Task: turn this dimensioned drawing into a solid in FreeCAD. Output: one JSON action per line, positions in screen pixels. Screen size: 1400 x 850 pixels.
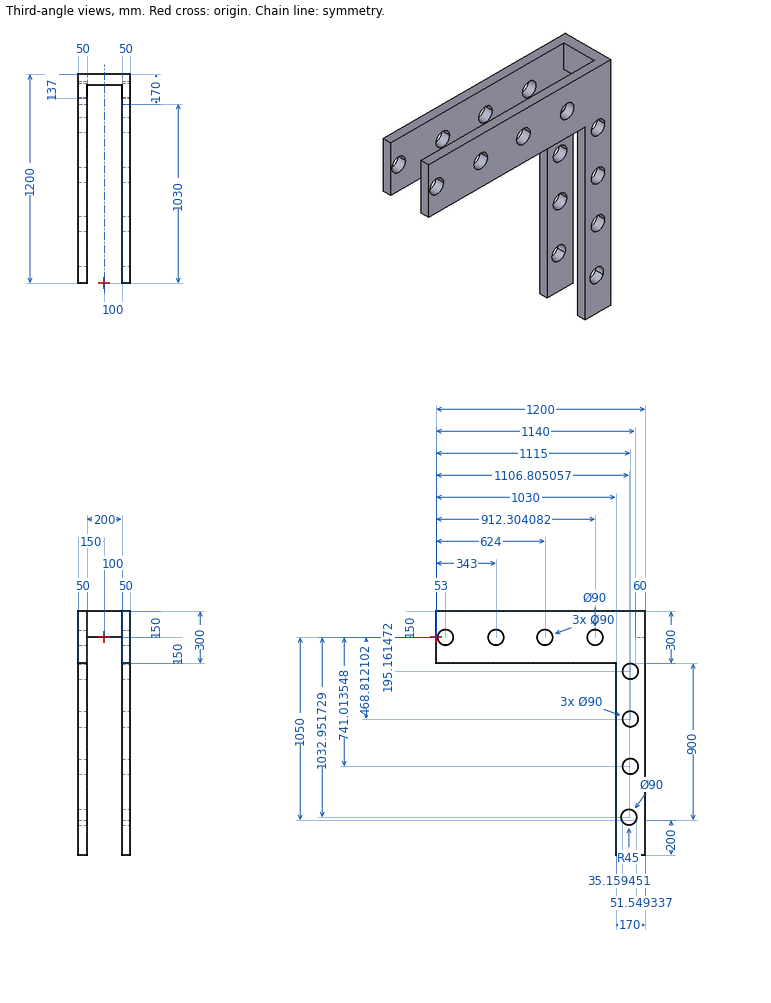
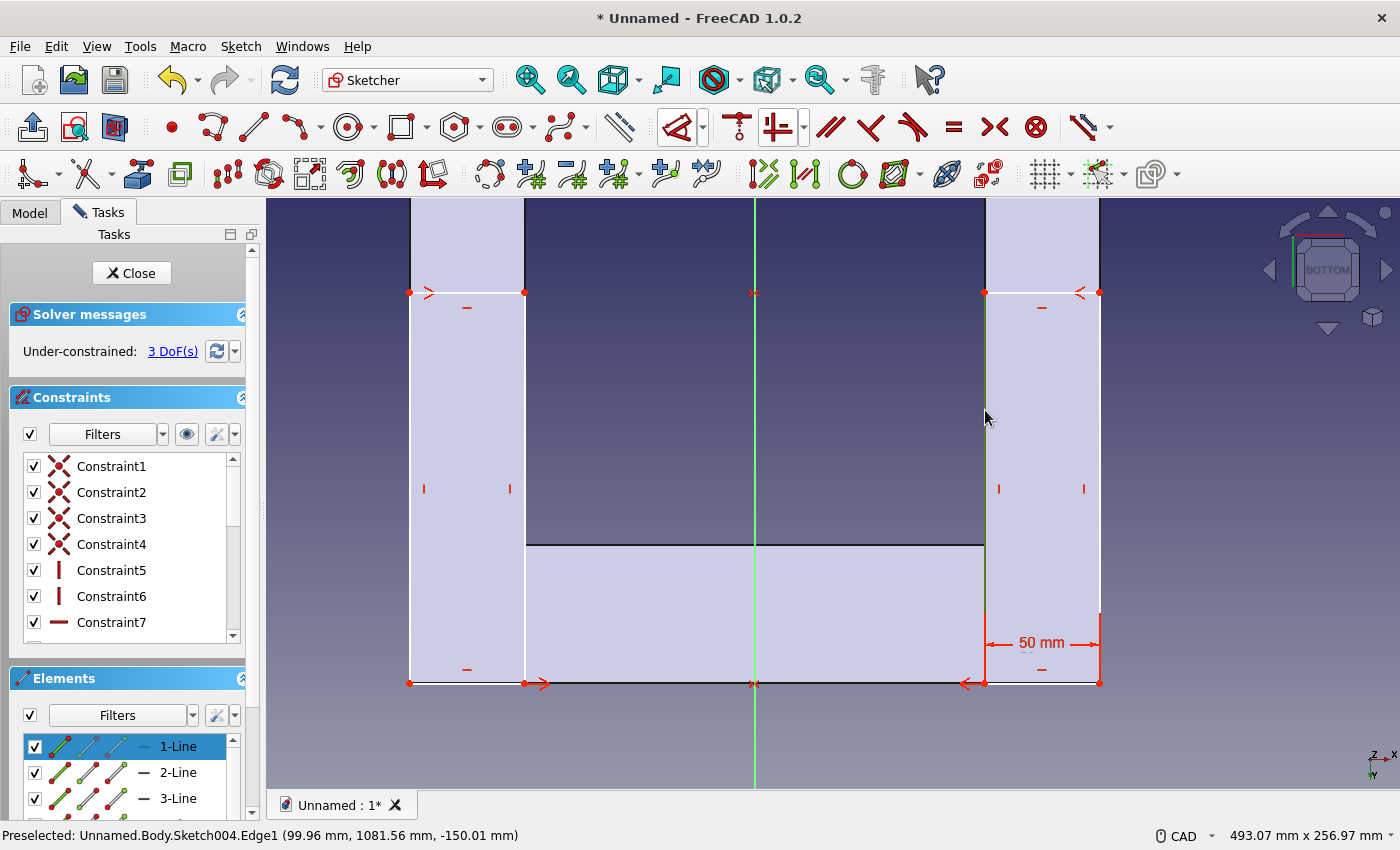
{"action": "key", "text": "i"}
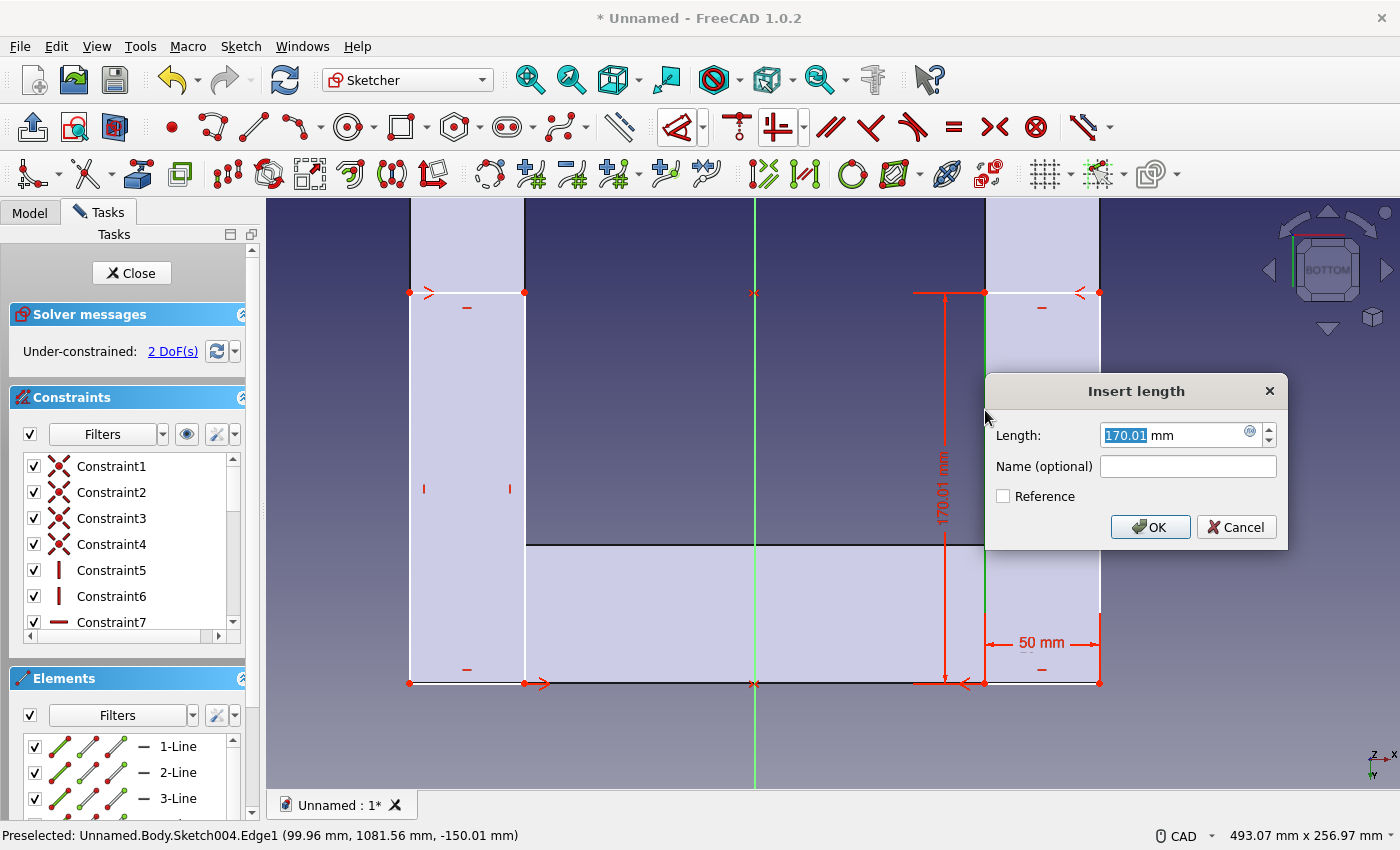
{"action": "type", "text": "170"}
{"action": "key", "text": "Return"}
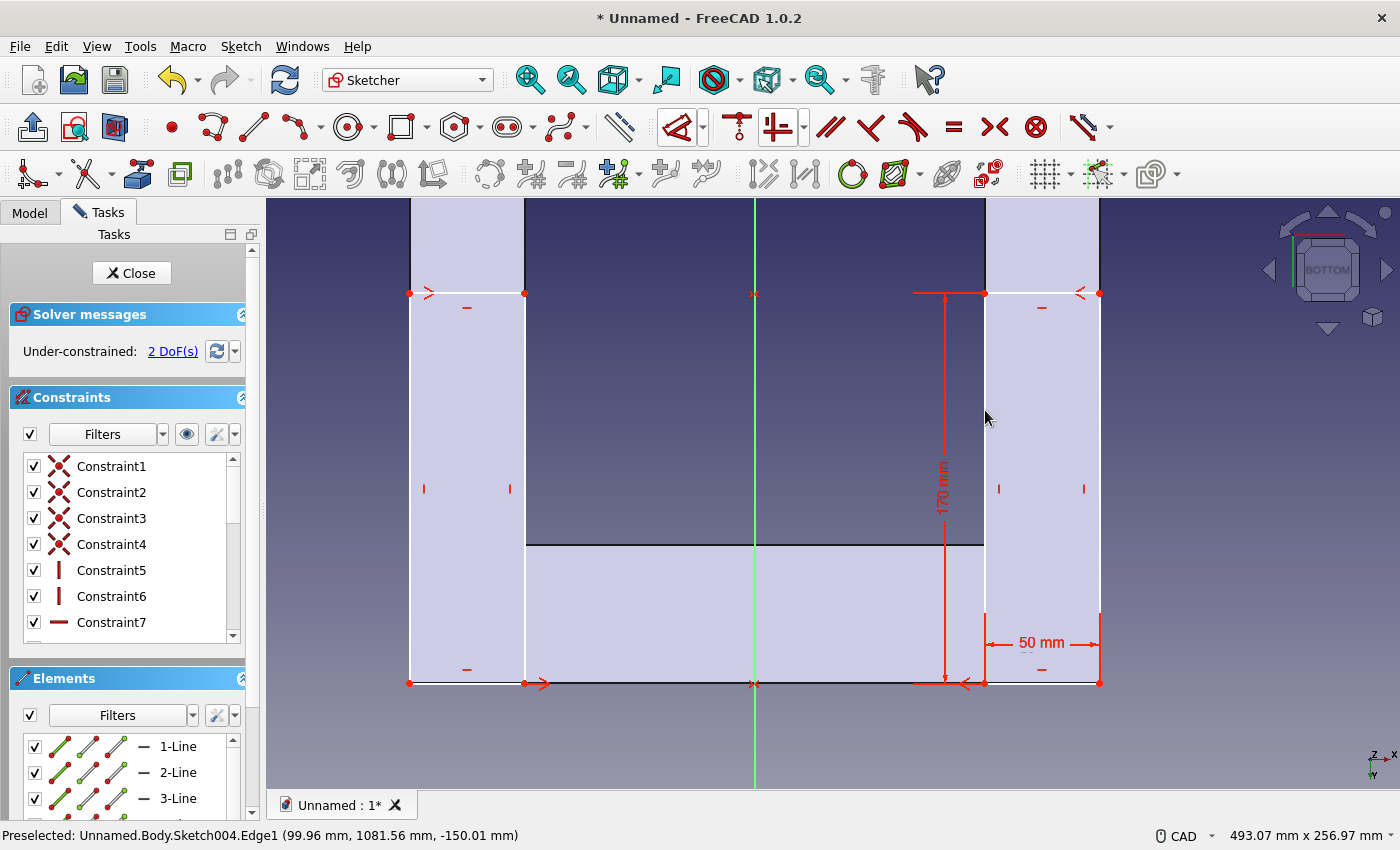
{"action": "left_click", "coordinate": [985, 293]}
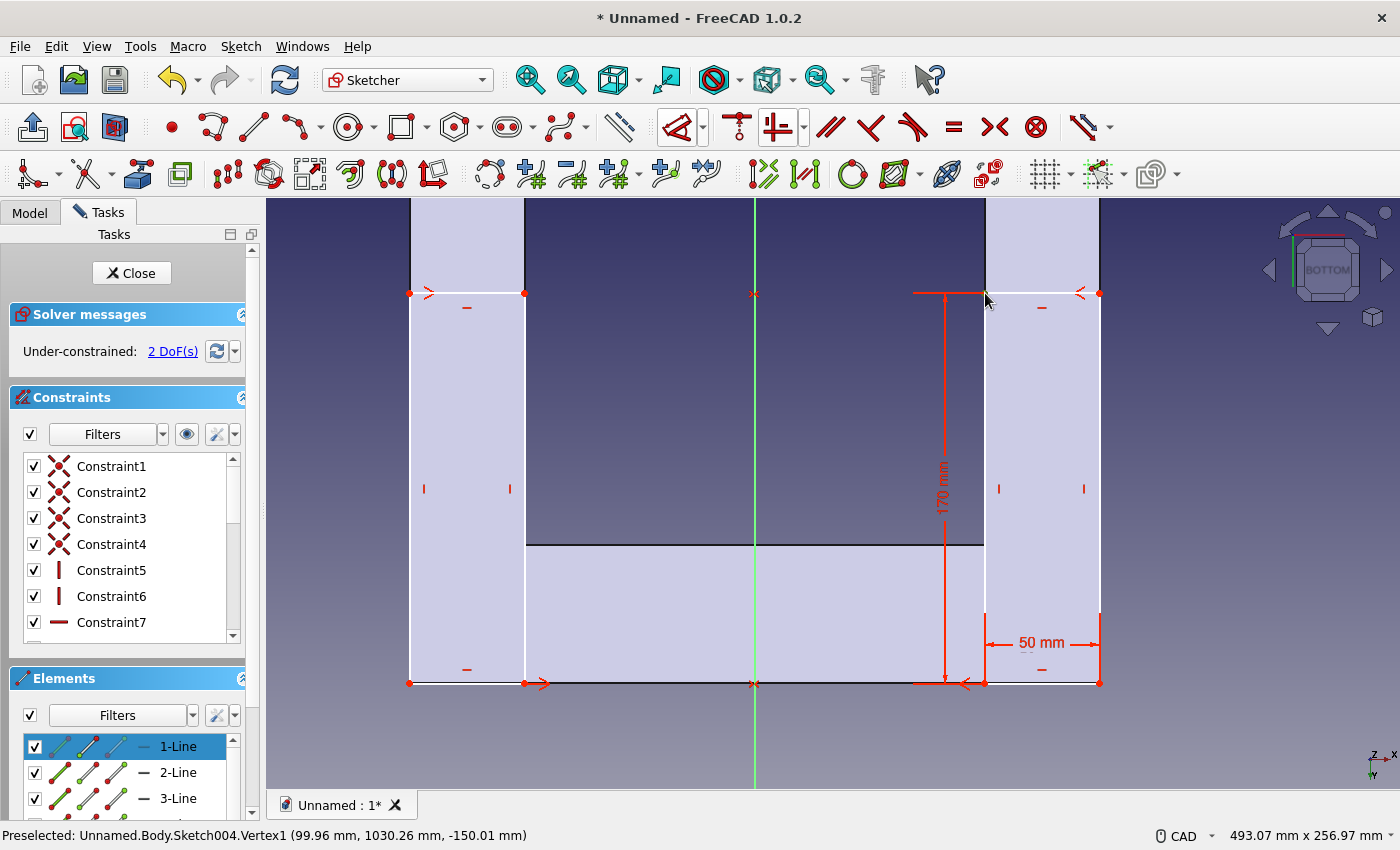
{"action": "key", "text": "l"}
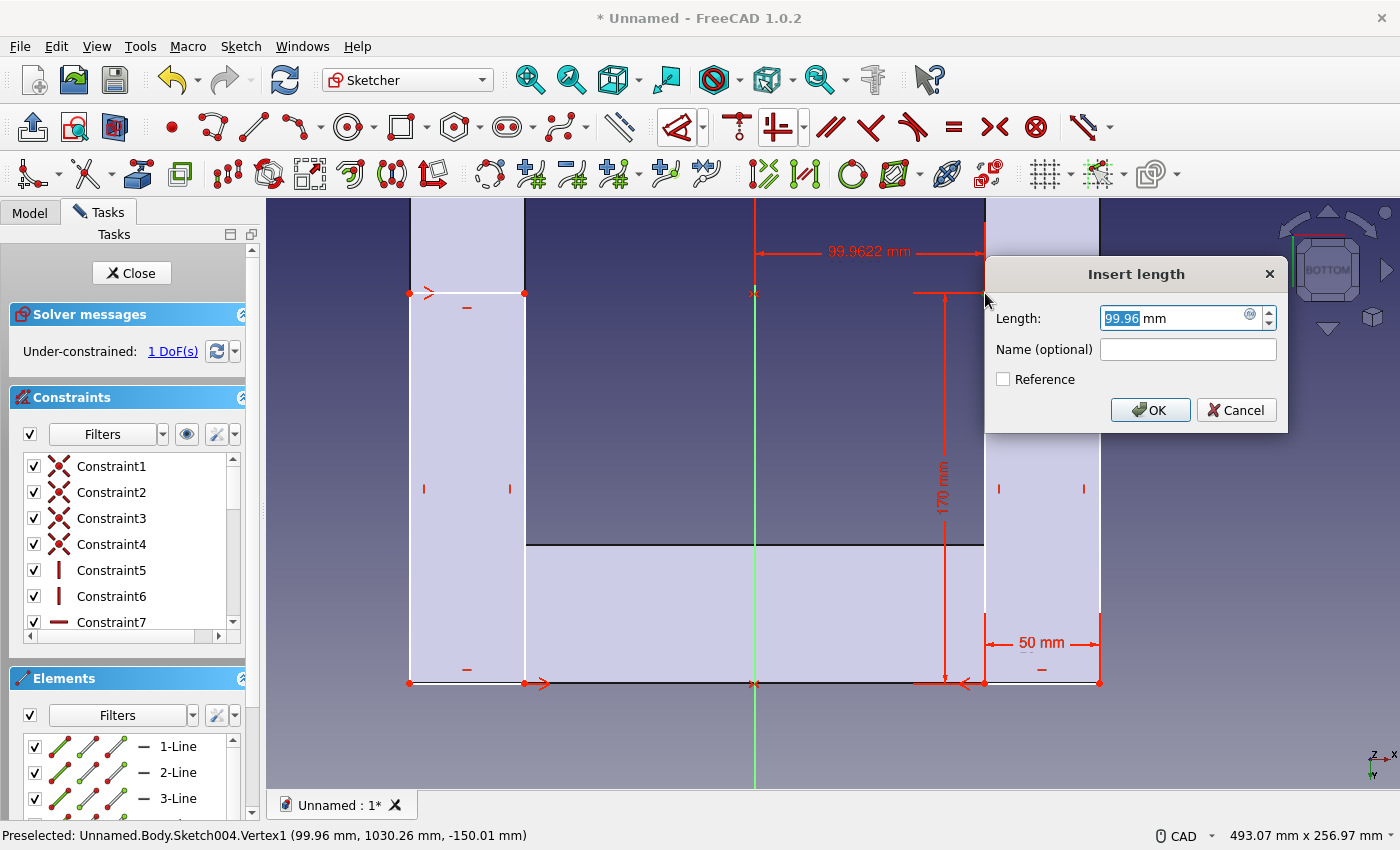
{"action": "type", "text": "100"}
{"action": "key", "text": "Return"}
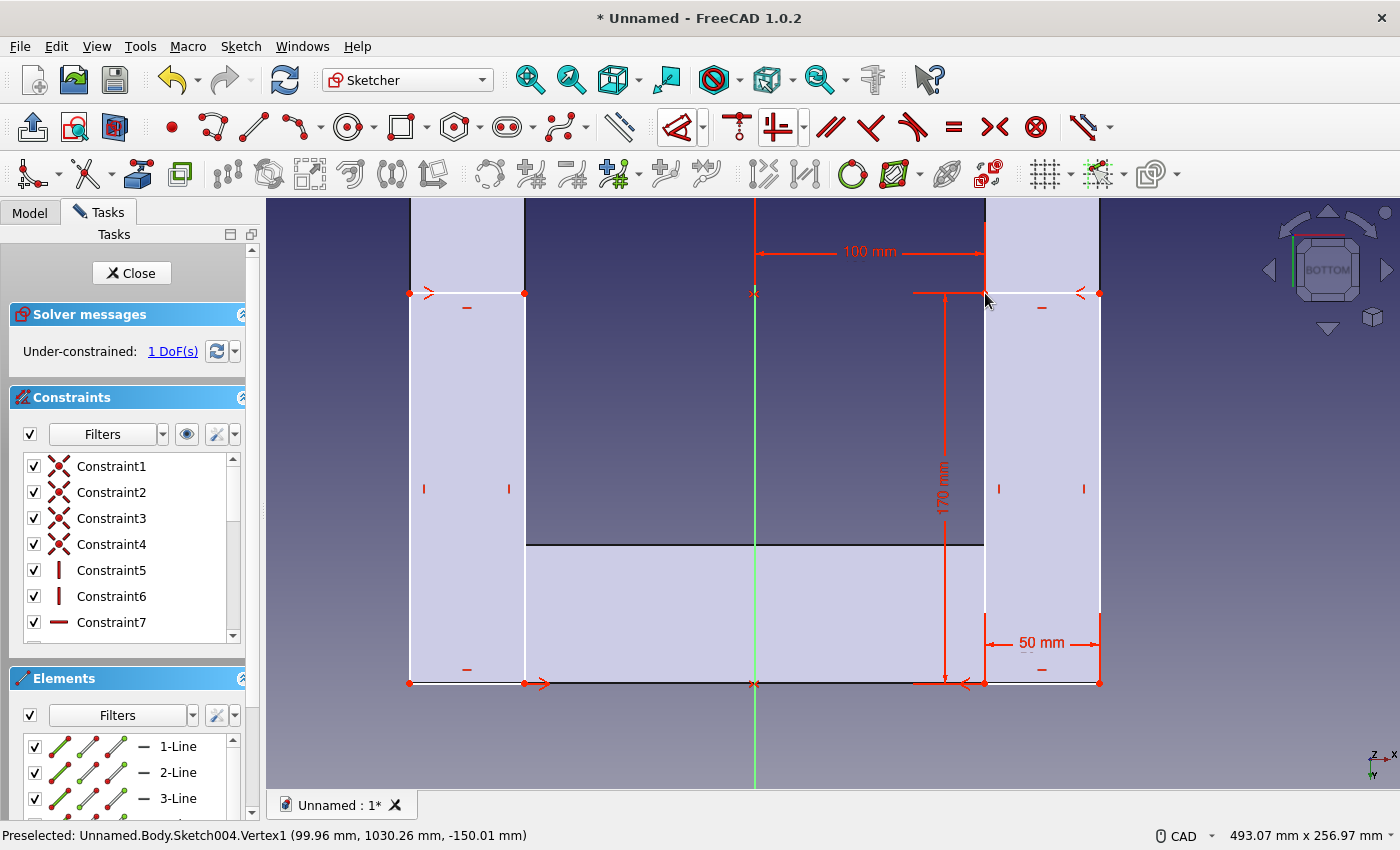
{"action": "left_click", "coordinate": [985, 293]}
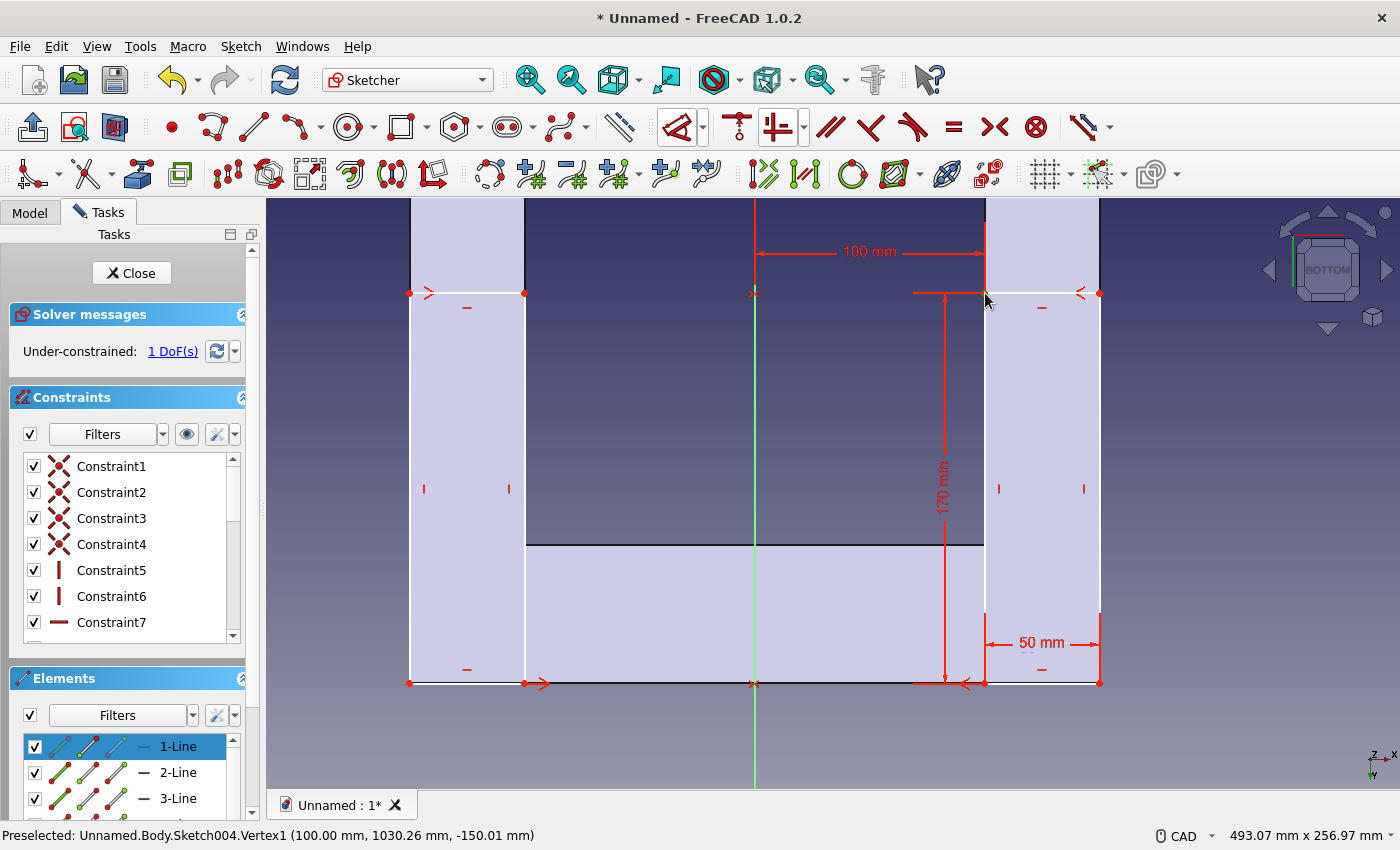
{"action": "left_click", "coordinate": [702, 128]}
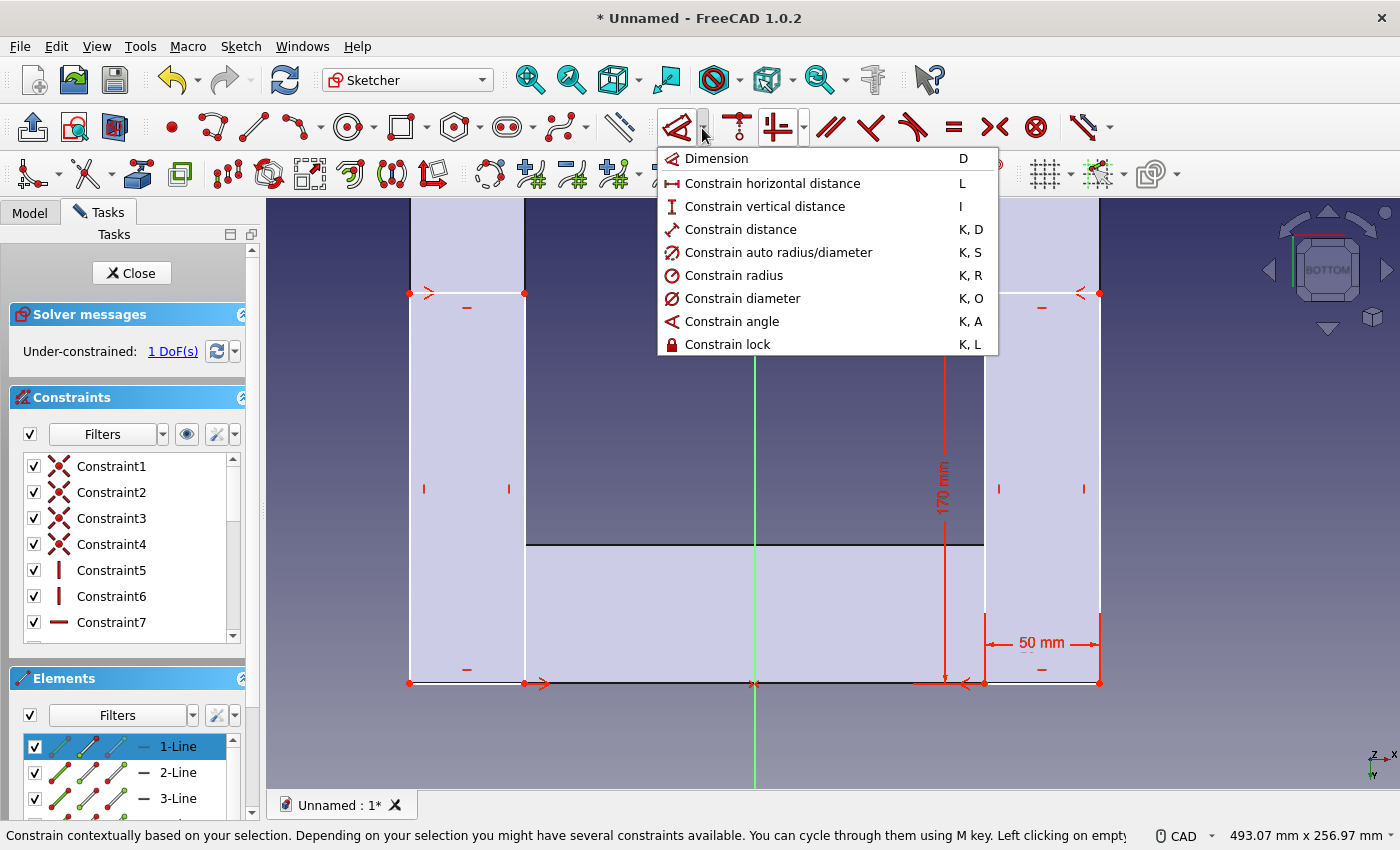
{"action": "left_click", "coordinate": [828, 206]}